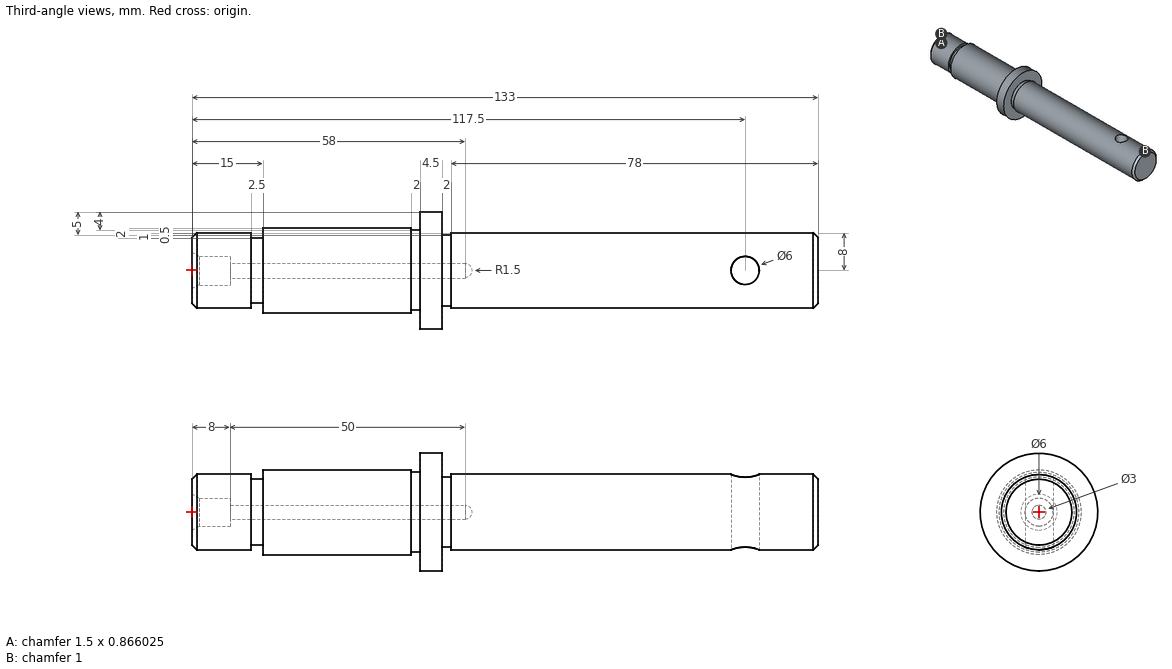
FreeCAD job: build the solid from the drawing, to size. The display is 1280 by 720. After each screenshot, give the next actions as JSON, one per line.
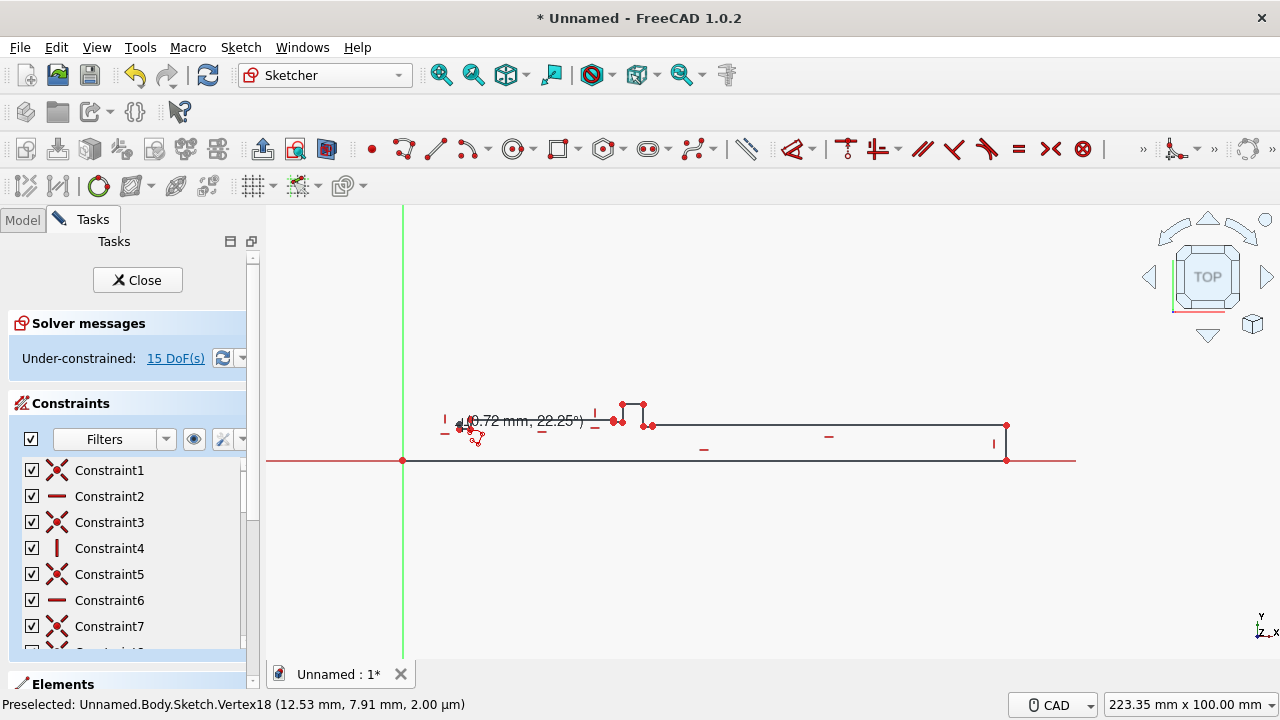
{"action": "left_click", "coordinate": [412, 424]}
{"action": "left_click", "coordinate": [403, 461]}
{"action": "key", "text": "Escape"}
{"action": "key", "text": "Escape"}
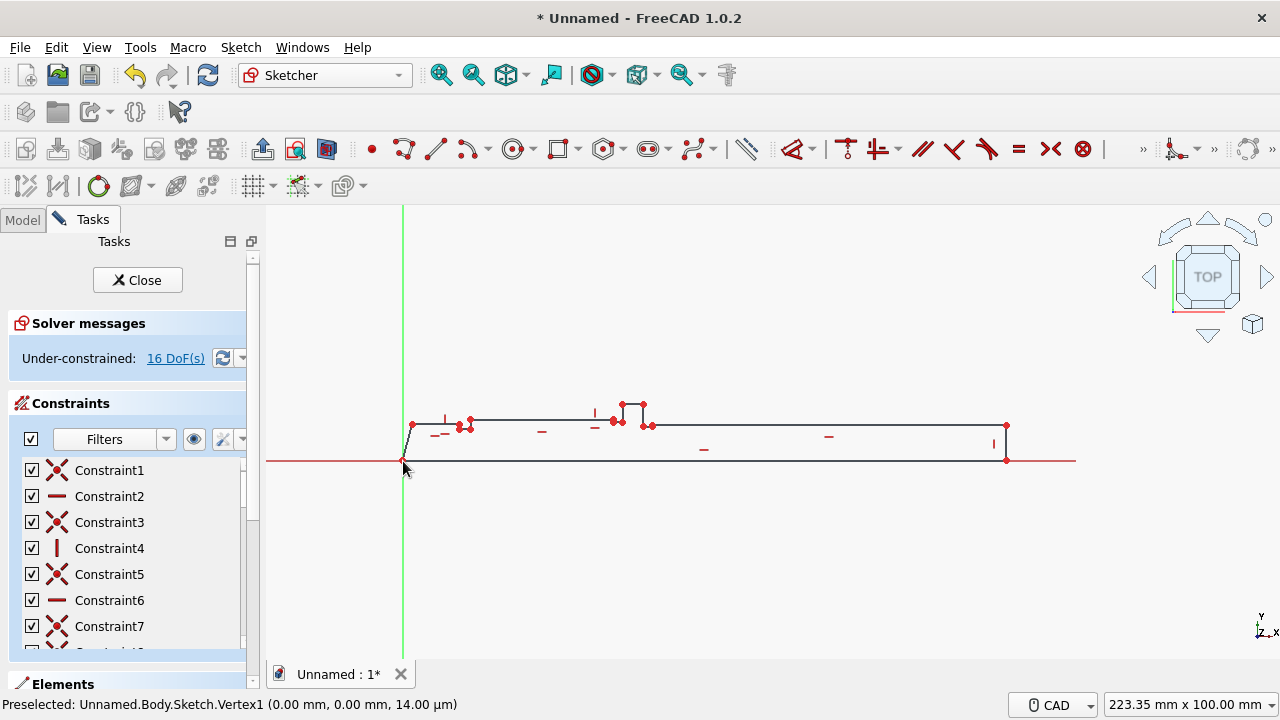
{"action": "scroll", "coordinate": [652, 426], "scroll_direction": "up", "scroll_amount": 14}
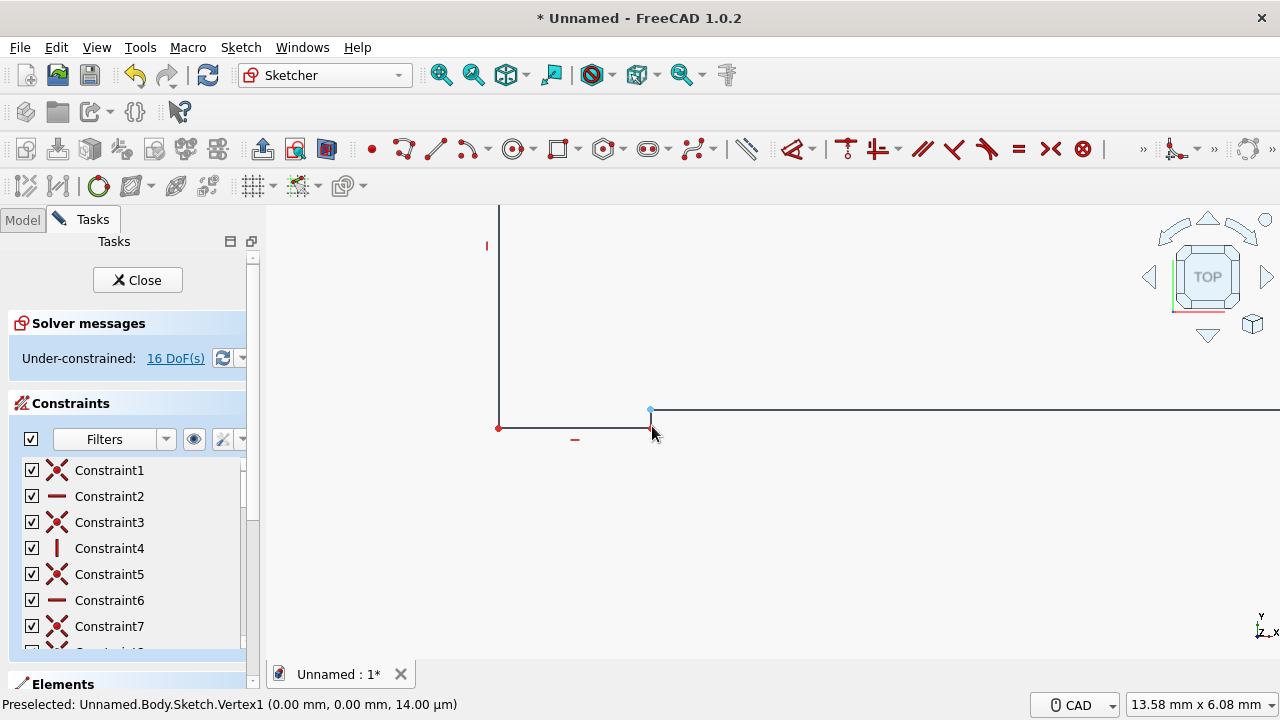
{"action": "left_click", "coordinate": [651, 419]}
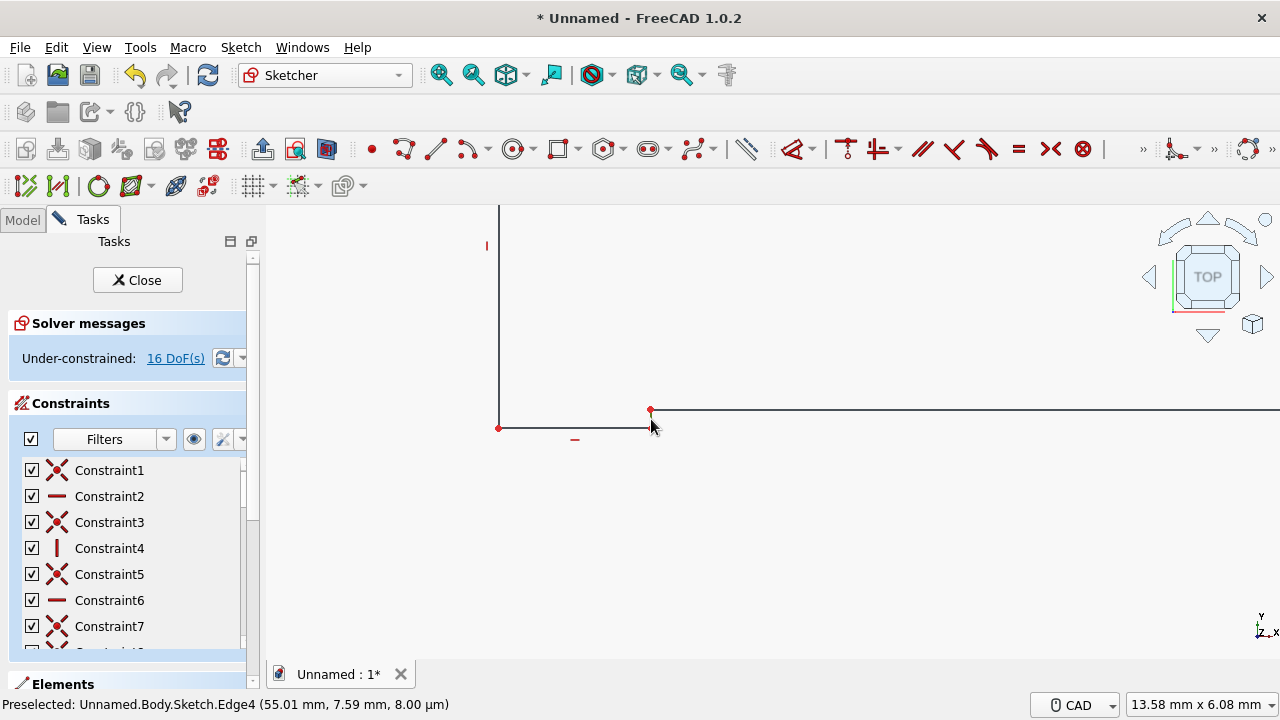
{"action": "key", "text": "v"}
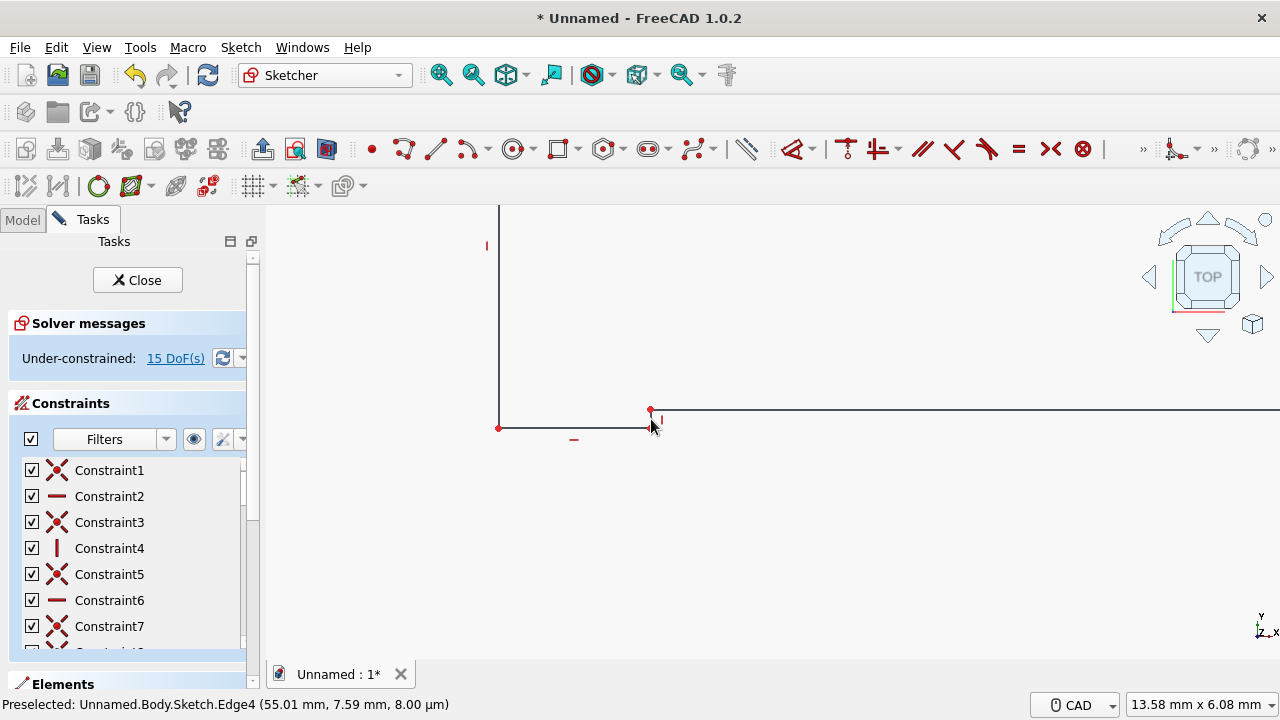
{"action": "scroll", "coordinate": [652, 426], "scroll_direction": "down", "scroll_amount": 14}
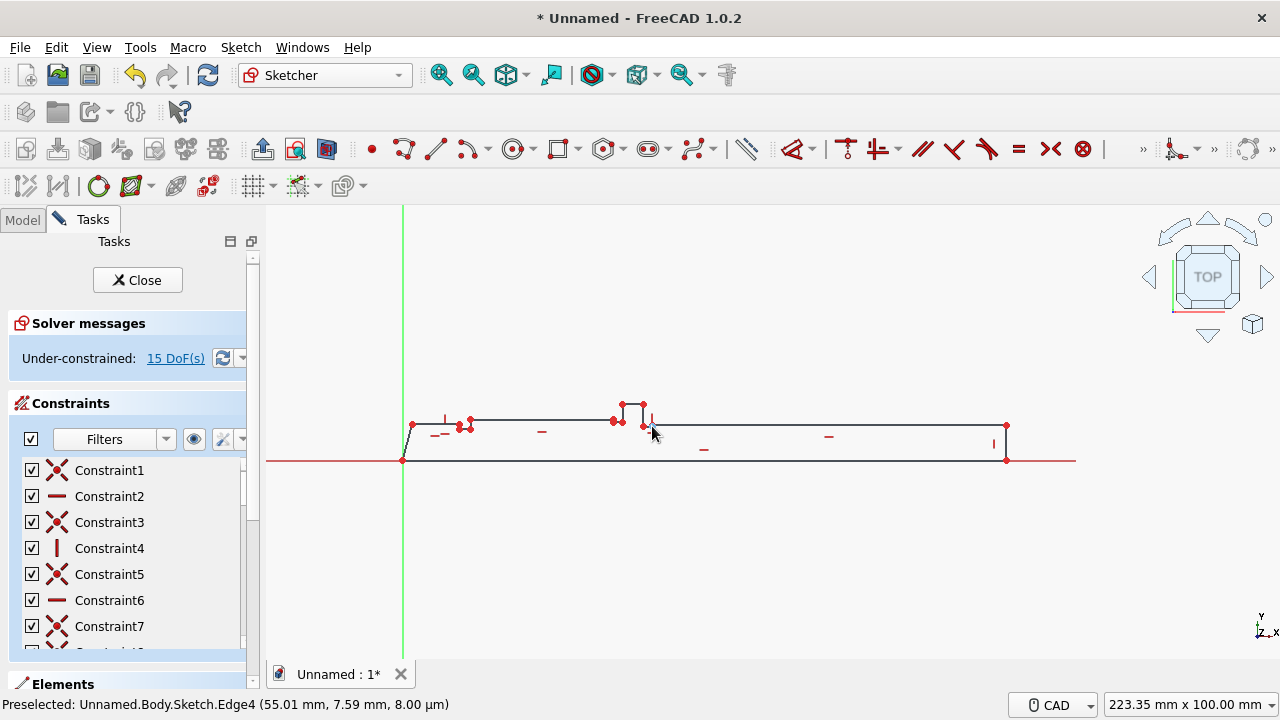
{"action": "scroll", "coordinate": [409, 435], "scroll_direction": "up", "scroll_amount": 4}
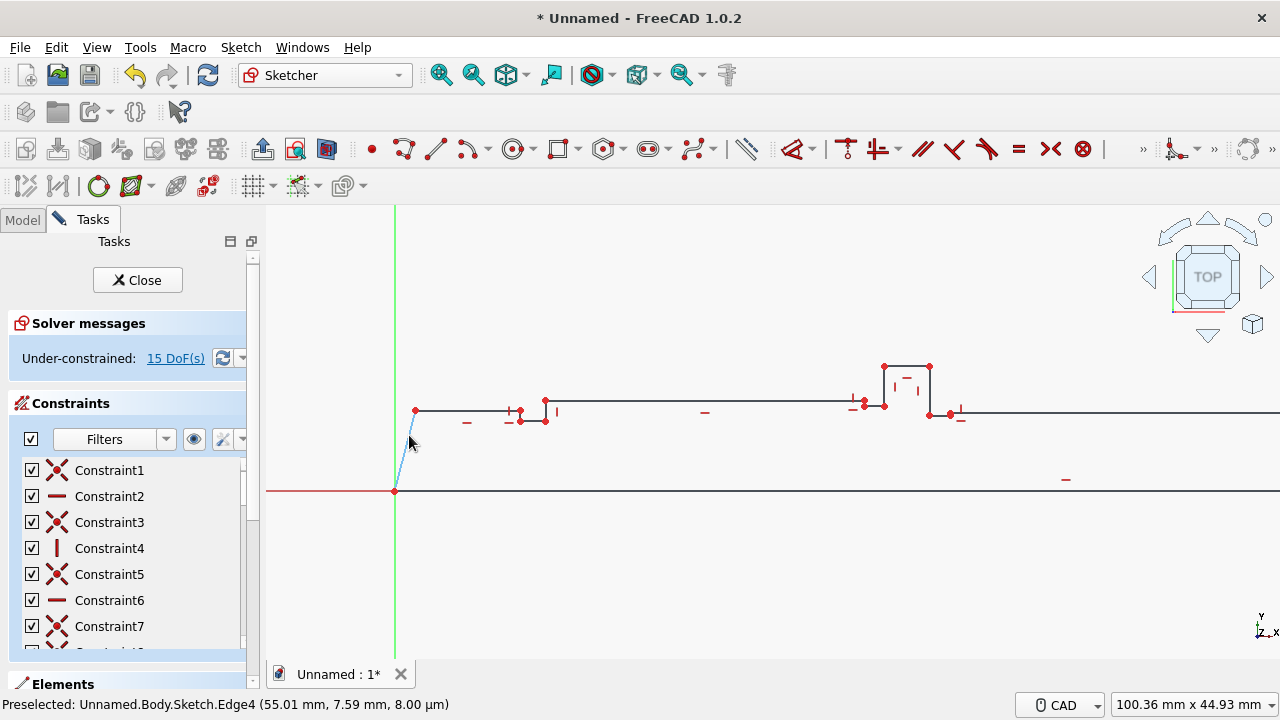
{"action": "left_click", "coordinate": [409, 435]}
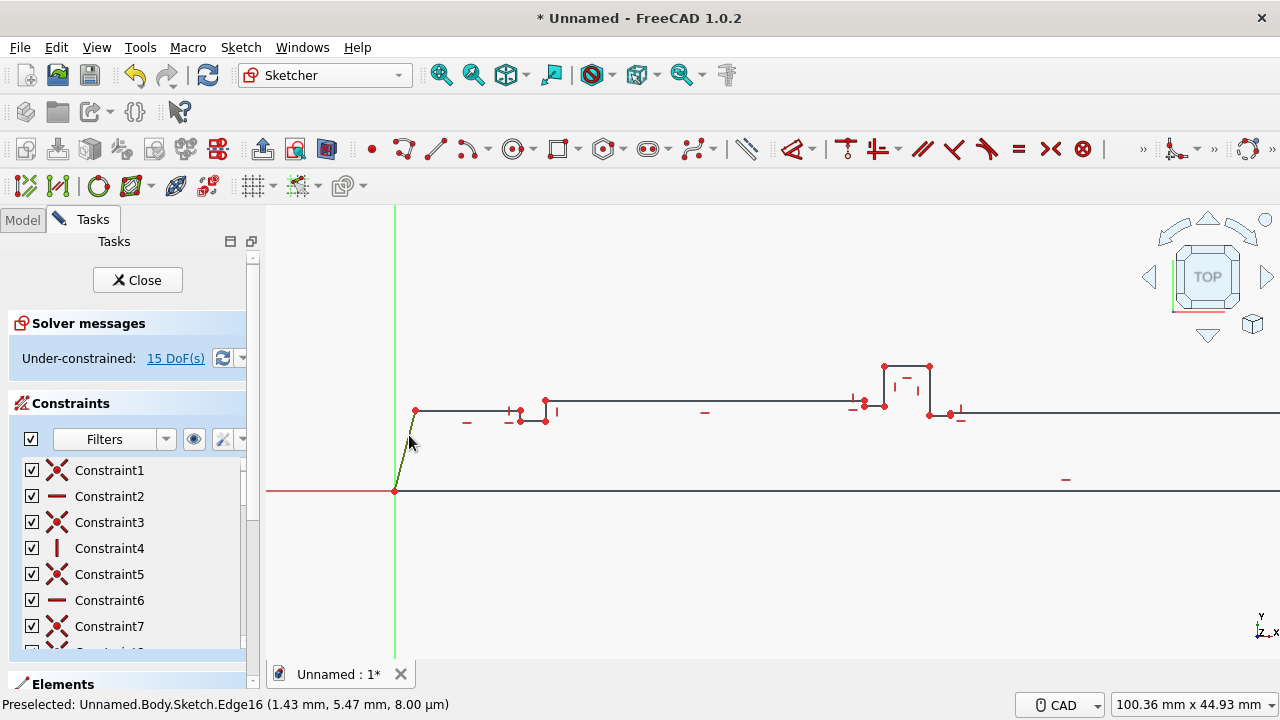
{"action": "key", "text": "v"}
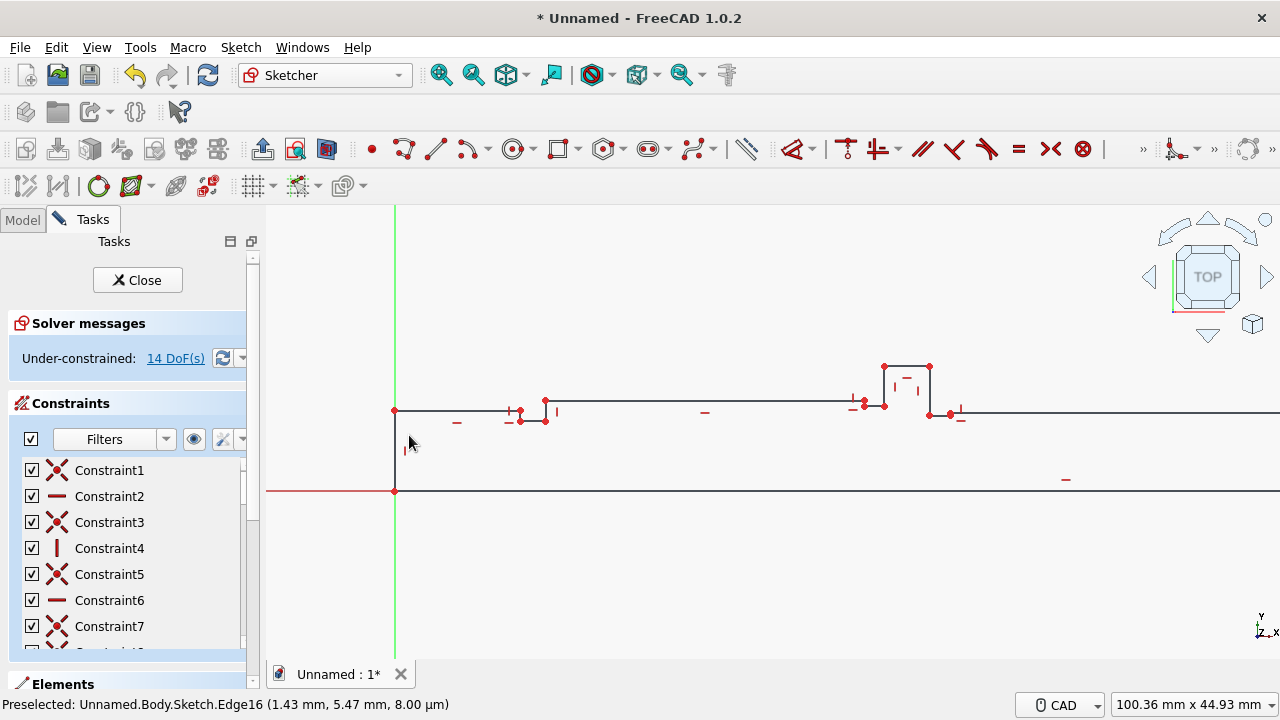
{"action": "scroll", "coordinate": [409, 435], "scroll_direction": "down", "scroll_amount": 4}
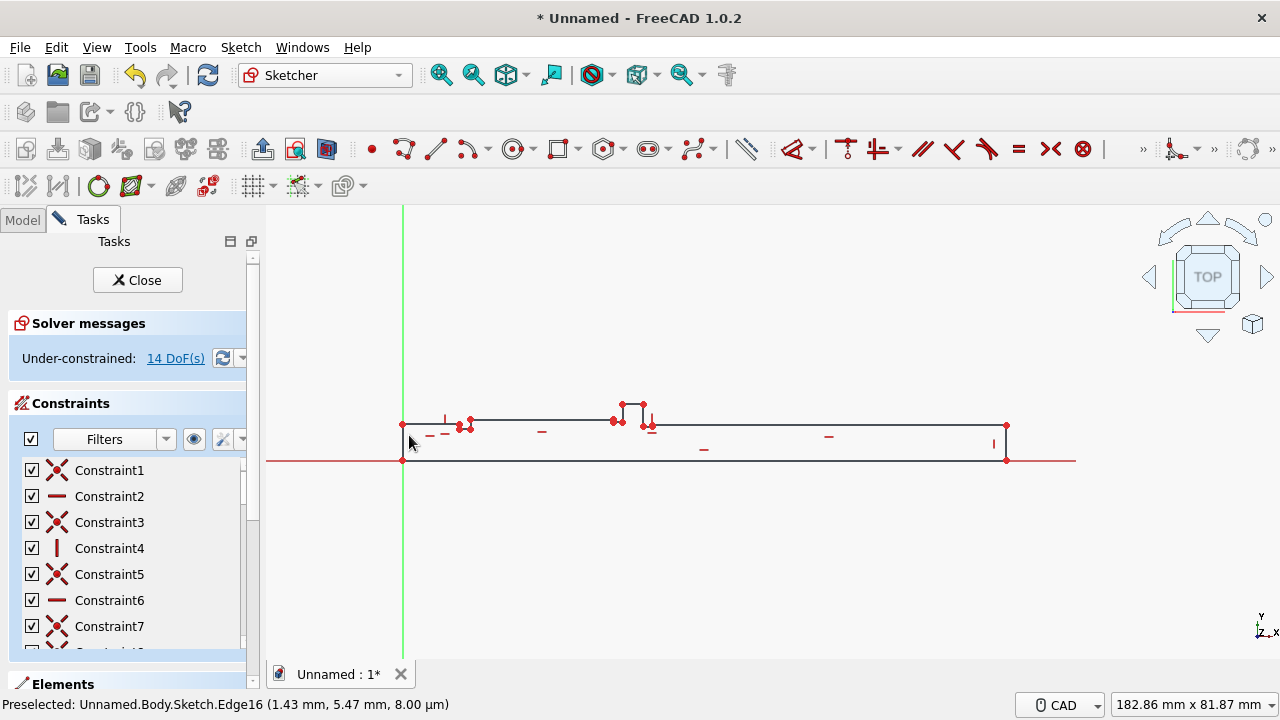
{"action": "scroll", "coordinate": [1006, 450], "scroll_direction": "up", "scroll_amount": 2}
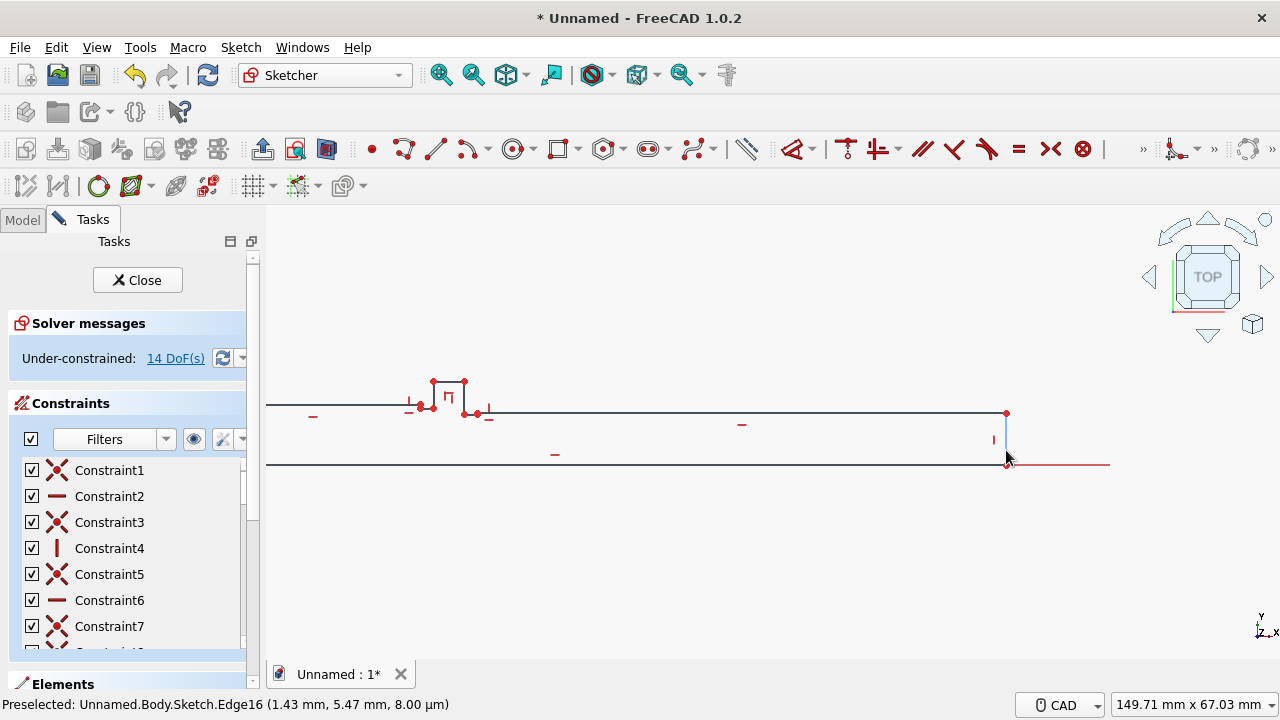
{"action": "left_click", "coordinate": [1006, 450]}